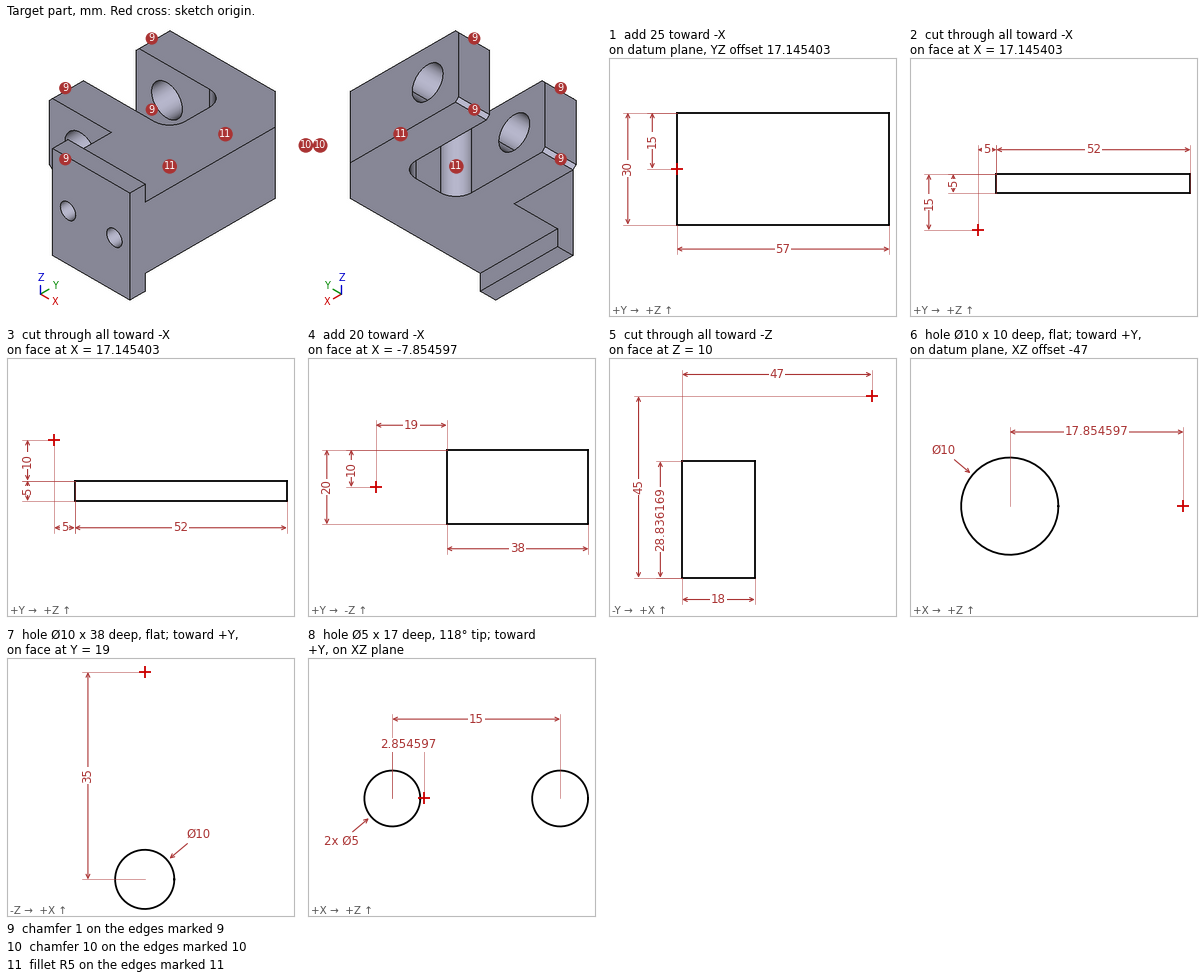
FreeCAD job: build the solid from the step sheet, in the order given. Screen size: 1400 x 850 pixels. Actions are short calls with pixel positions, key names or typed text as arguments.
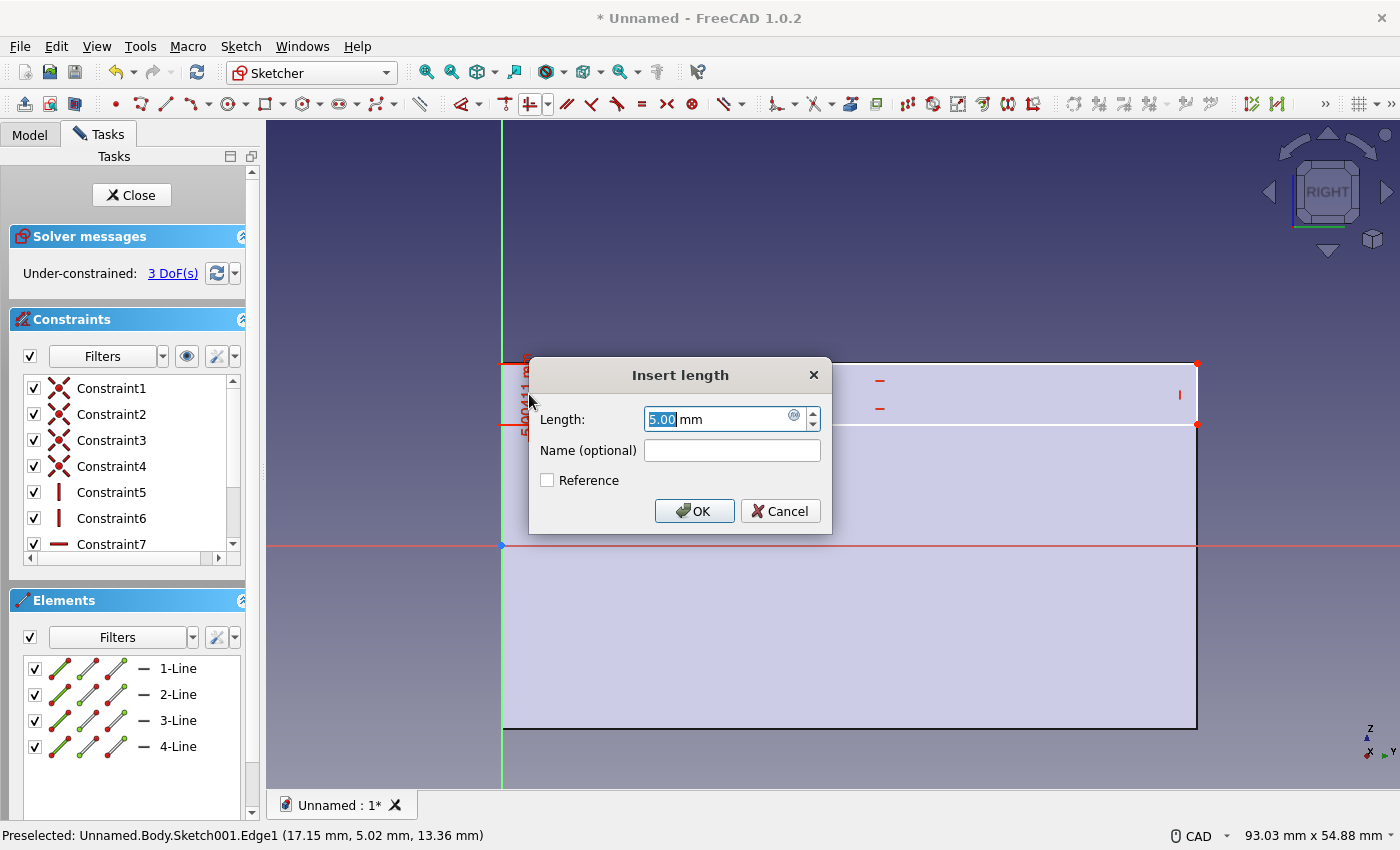
text(5)
key(Return)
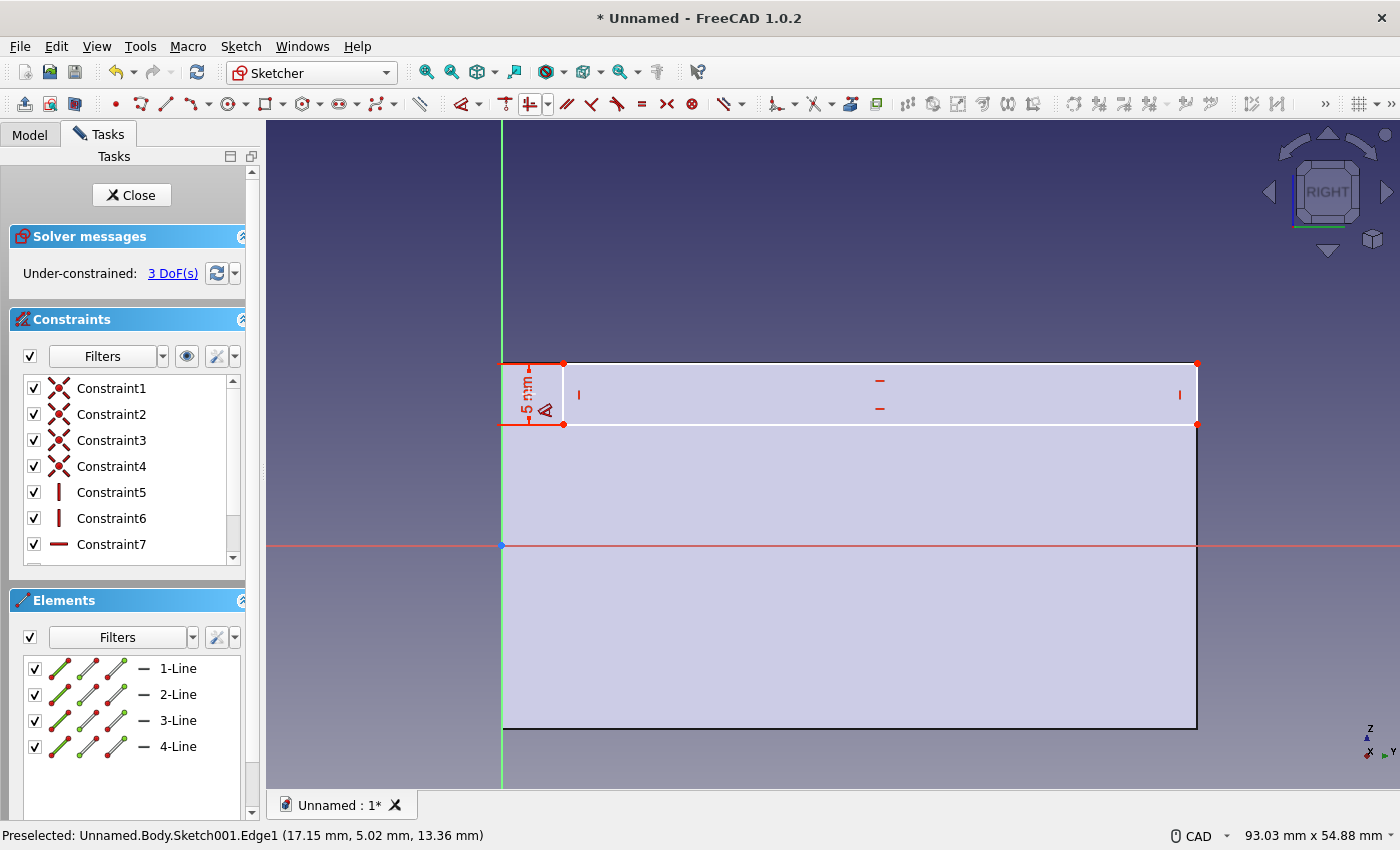
click(753, 425)
click(880, 391)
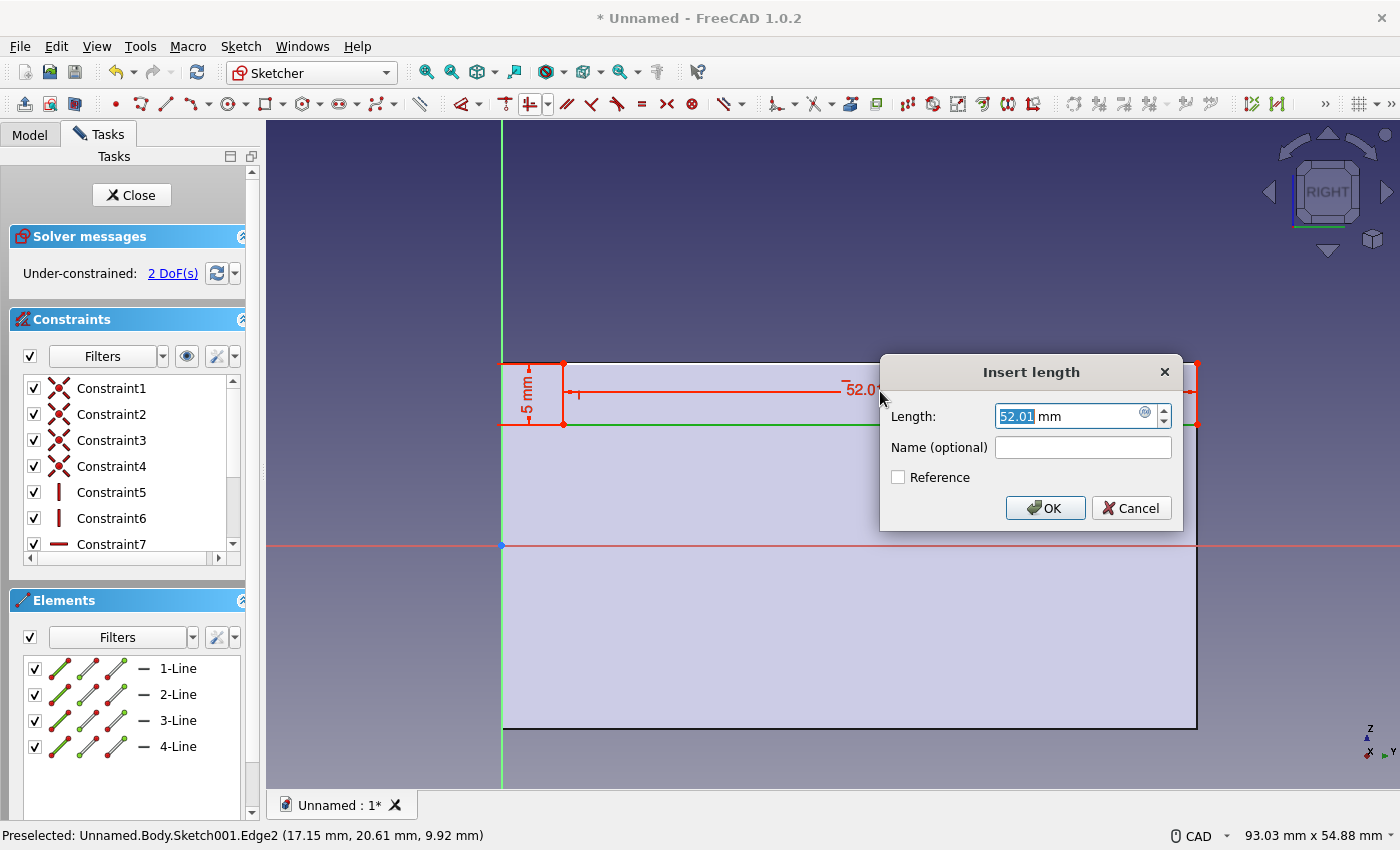
text(52)
key(Return)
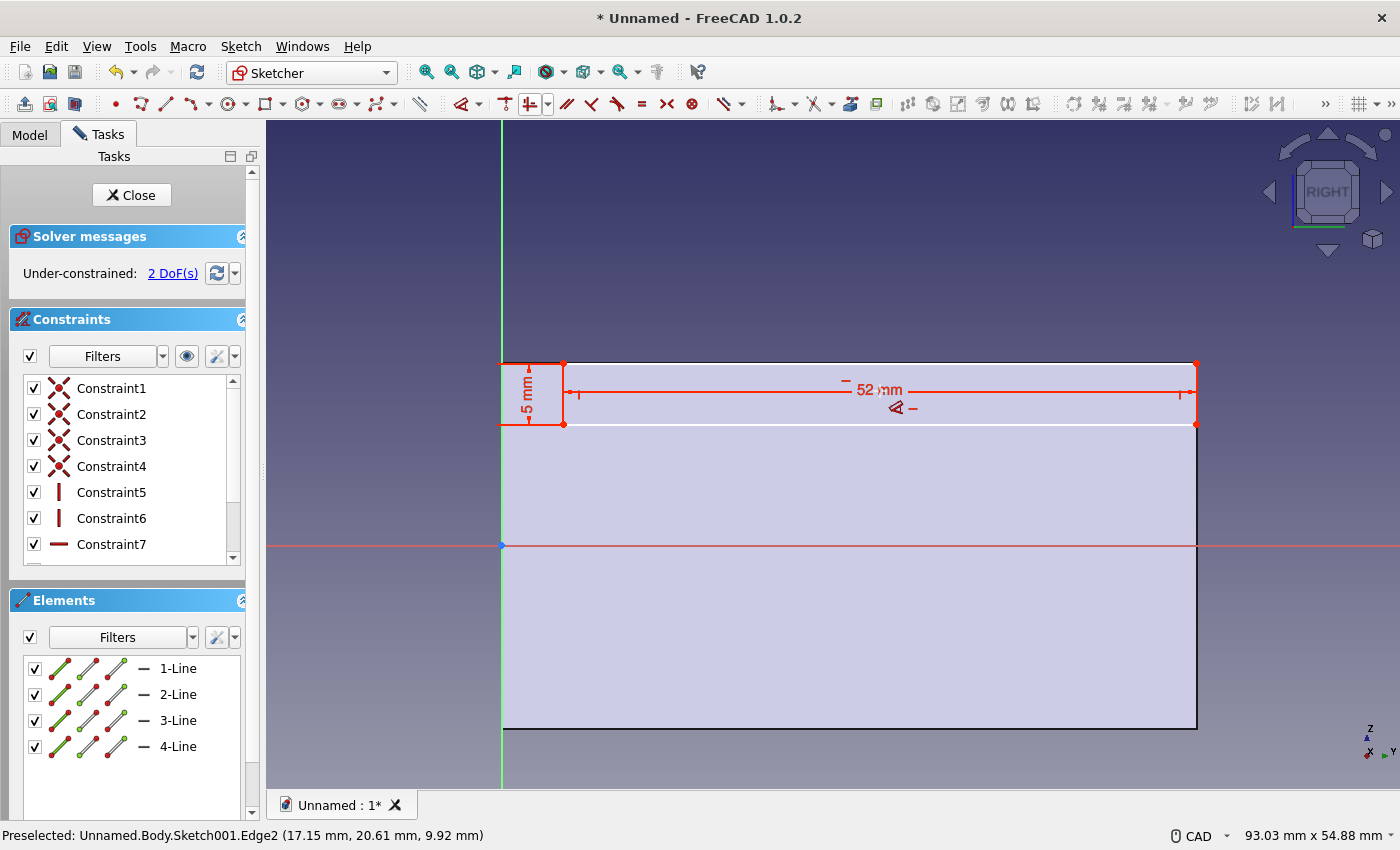
click(563, 364)
click(532, 580)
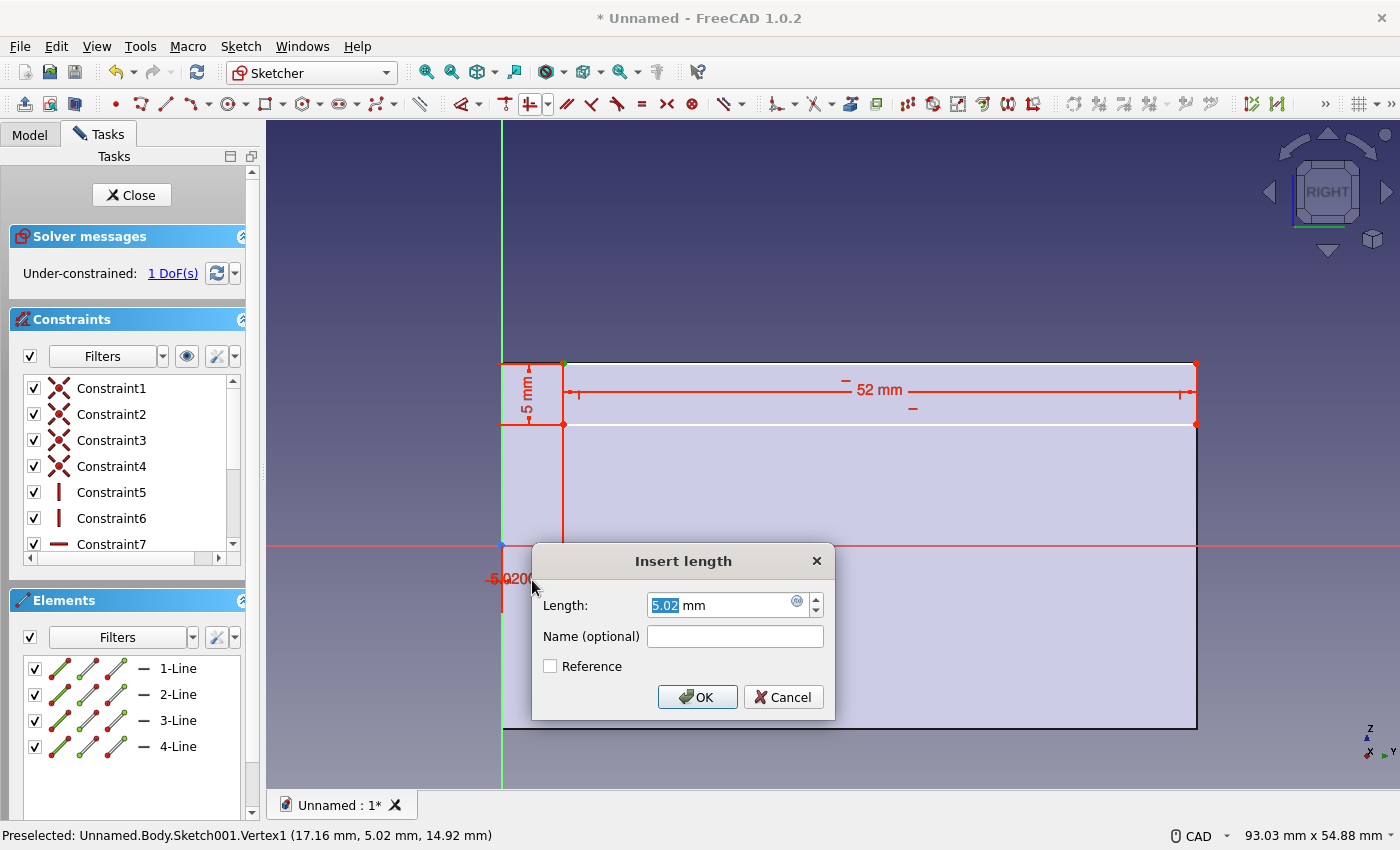
text(5)
key(Return)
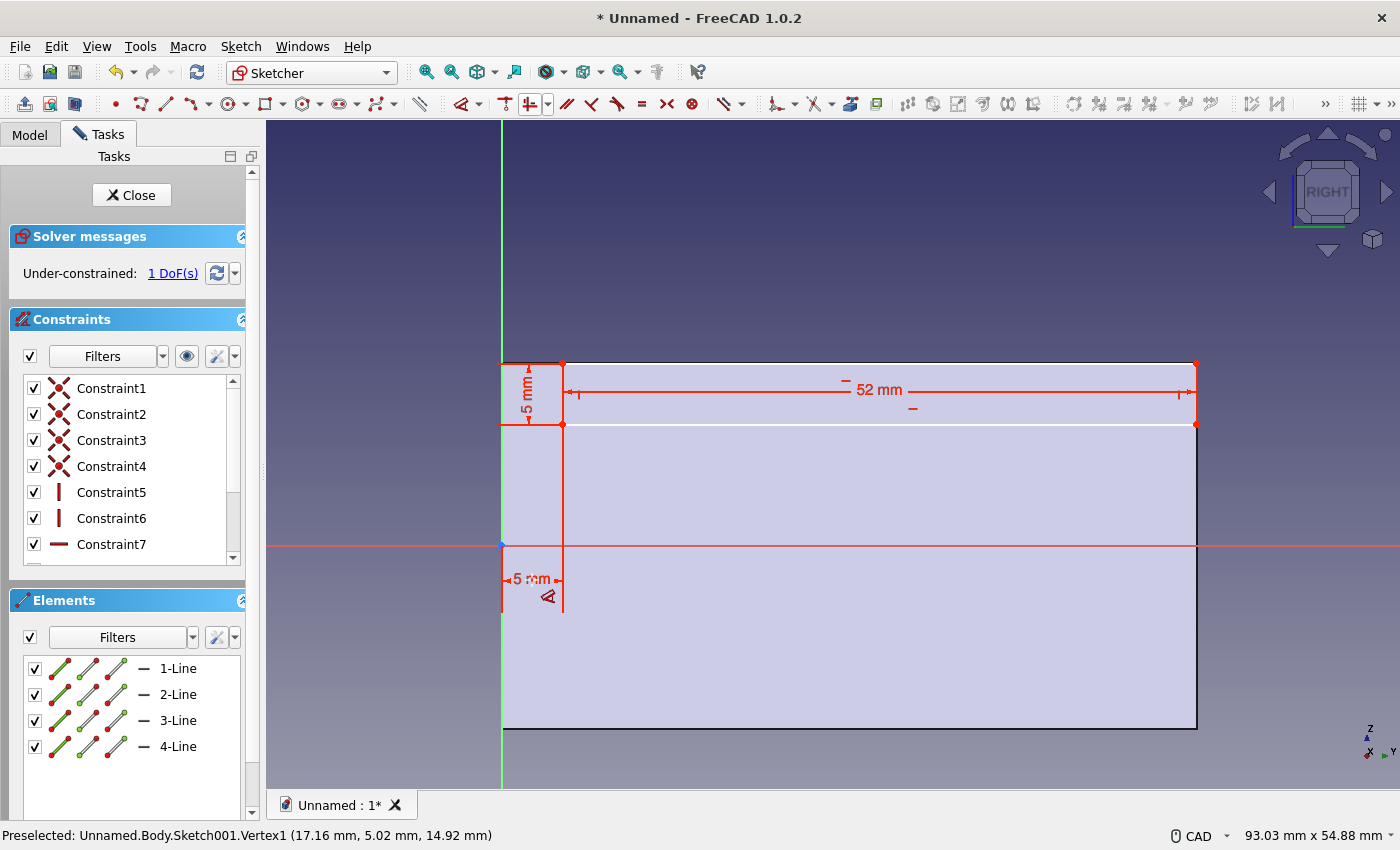
click(563, 364)
click(468, 455)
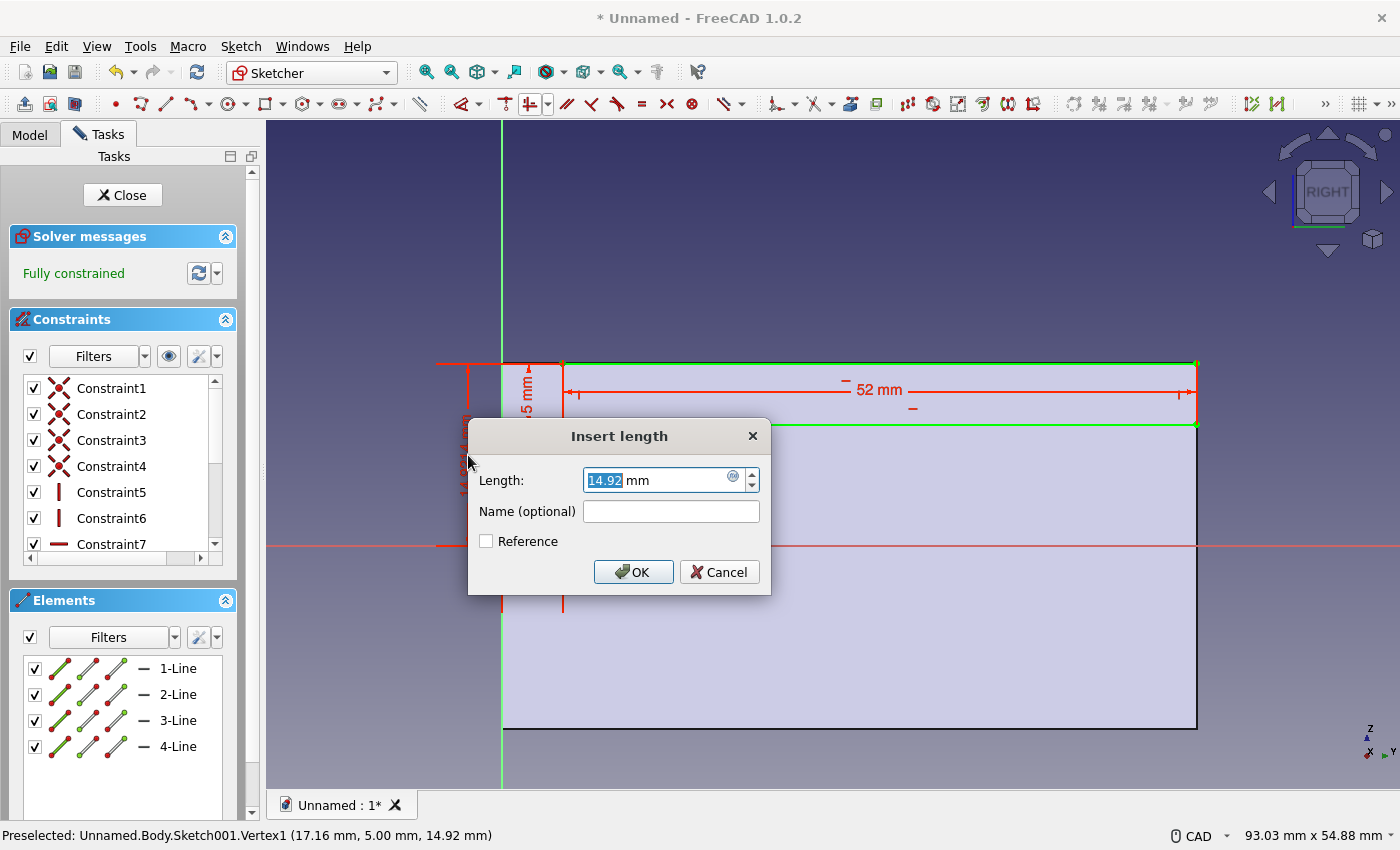
text(15)
key(Return)
key(Escape)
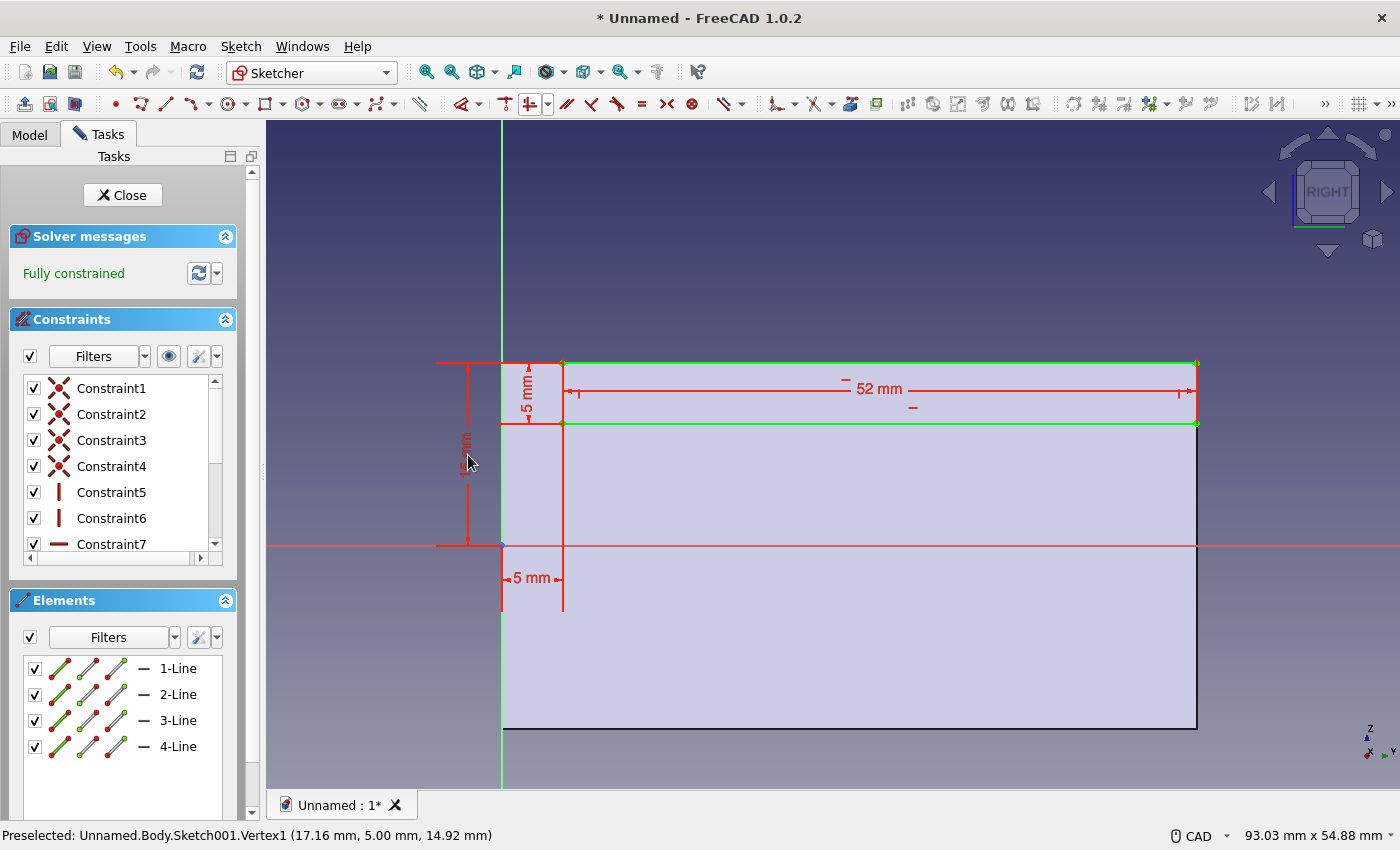
click(123, 195)